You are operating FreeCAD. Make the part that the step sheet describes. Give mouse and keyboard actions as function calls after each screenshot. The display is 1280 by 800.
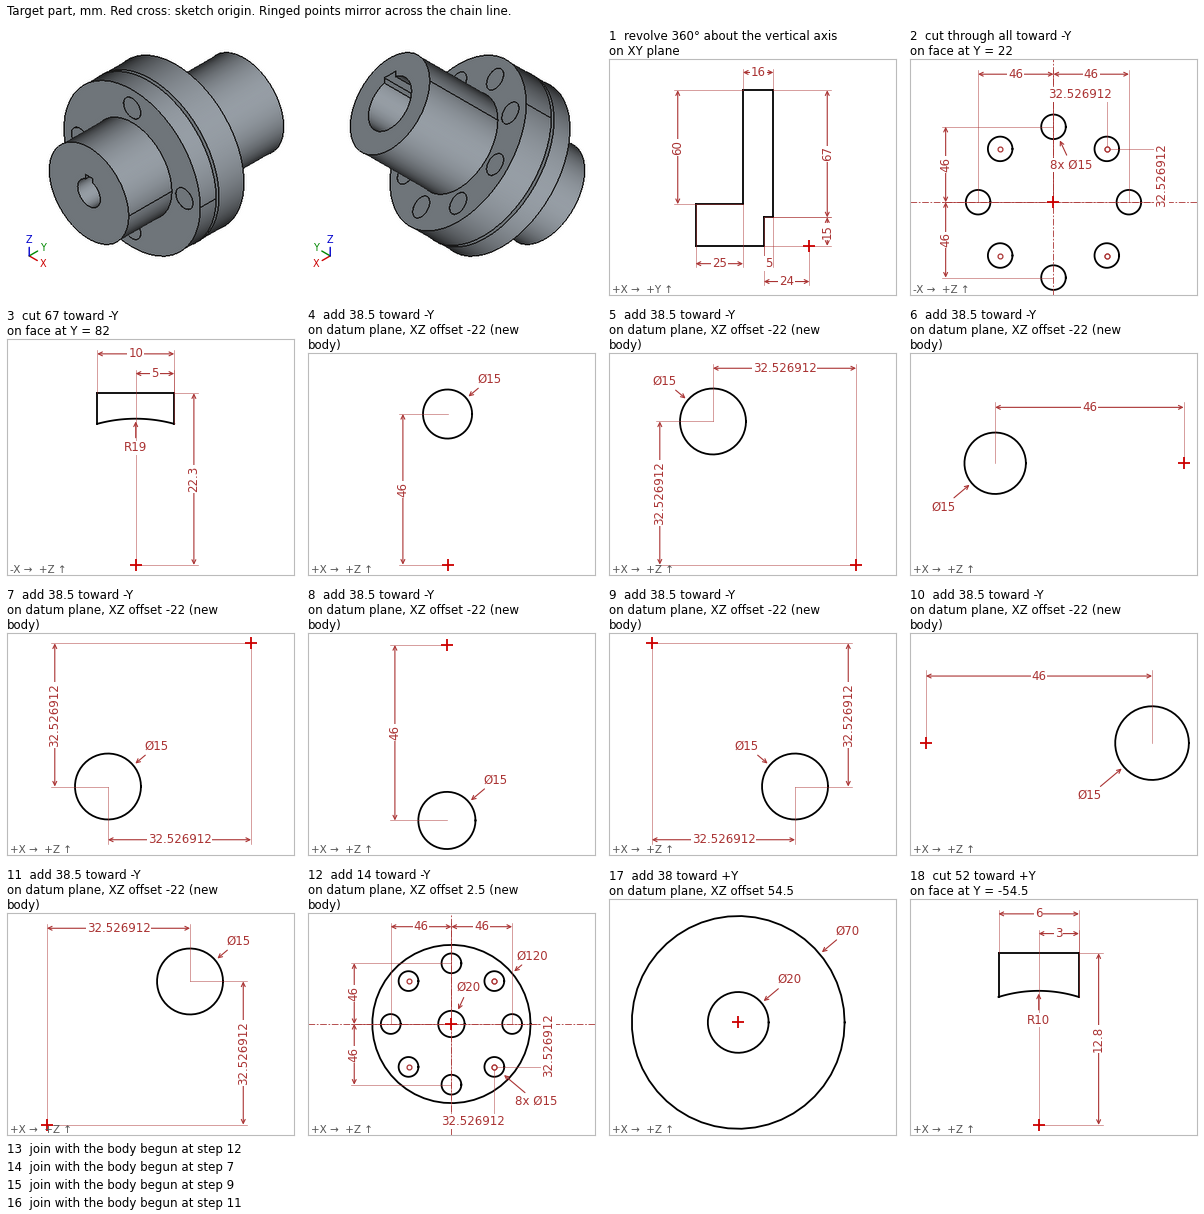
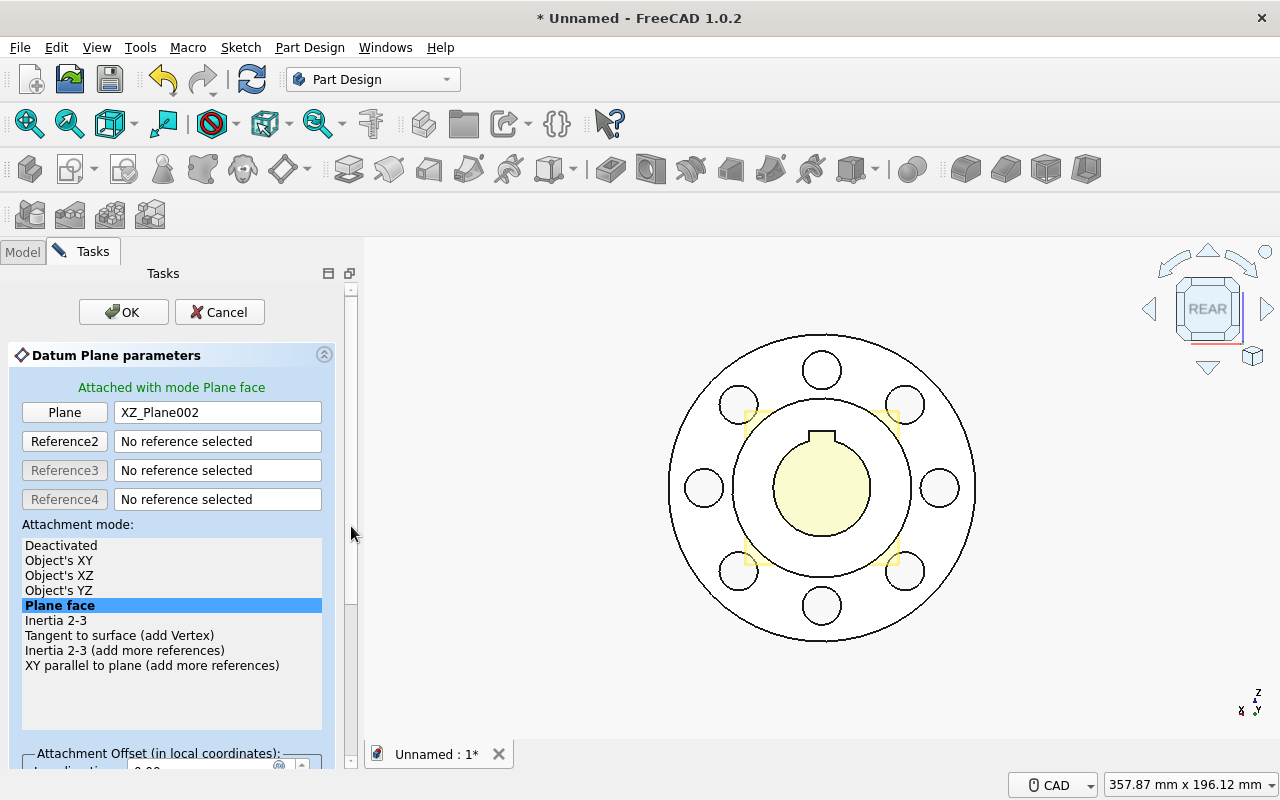
click(124, 312)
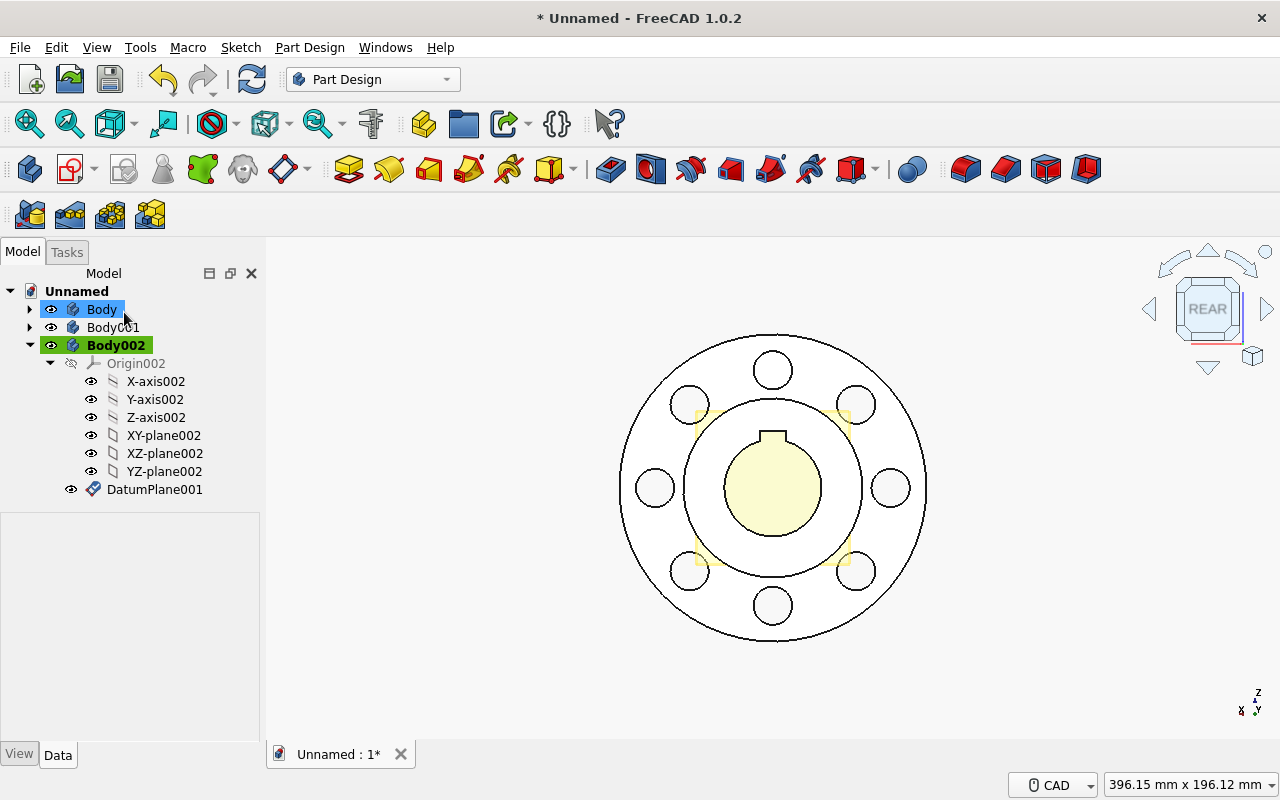
click(116, 489)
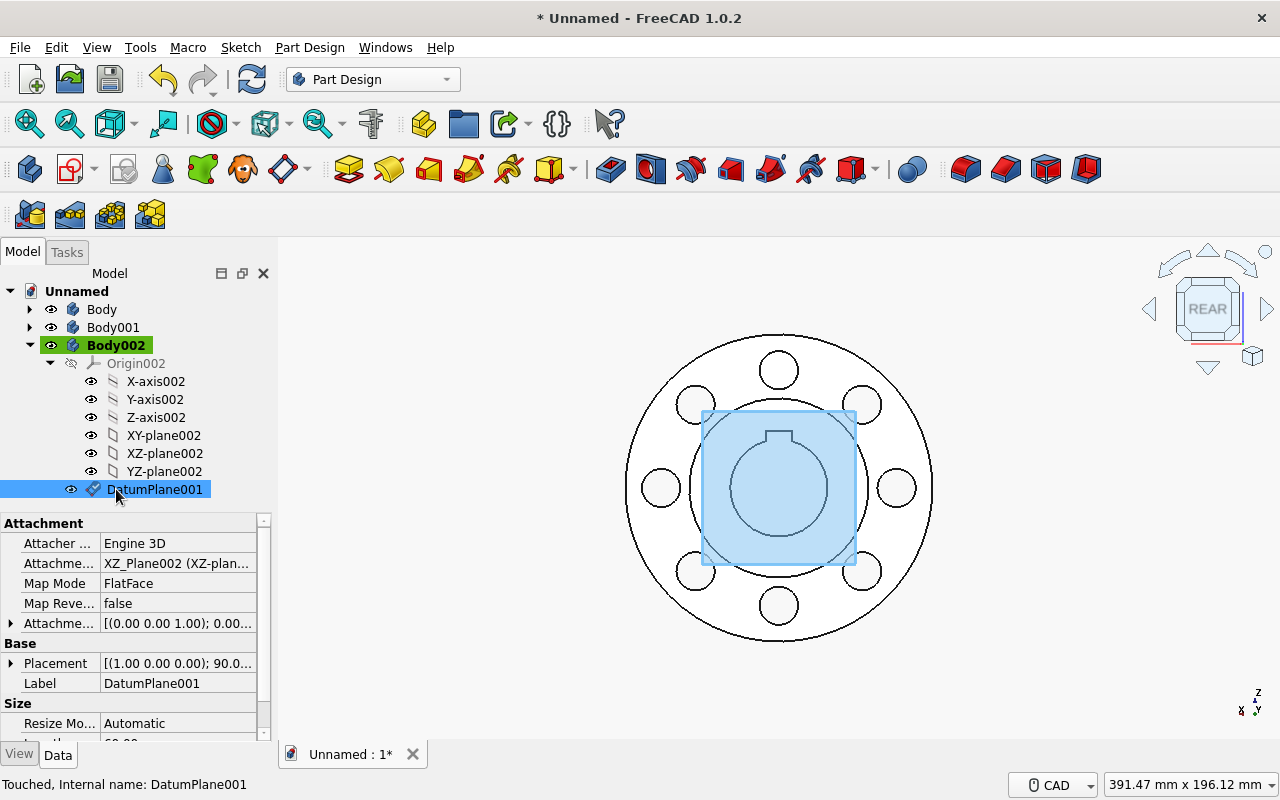
click(70, 170)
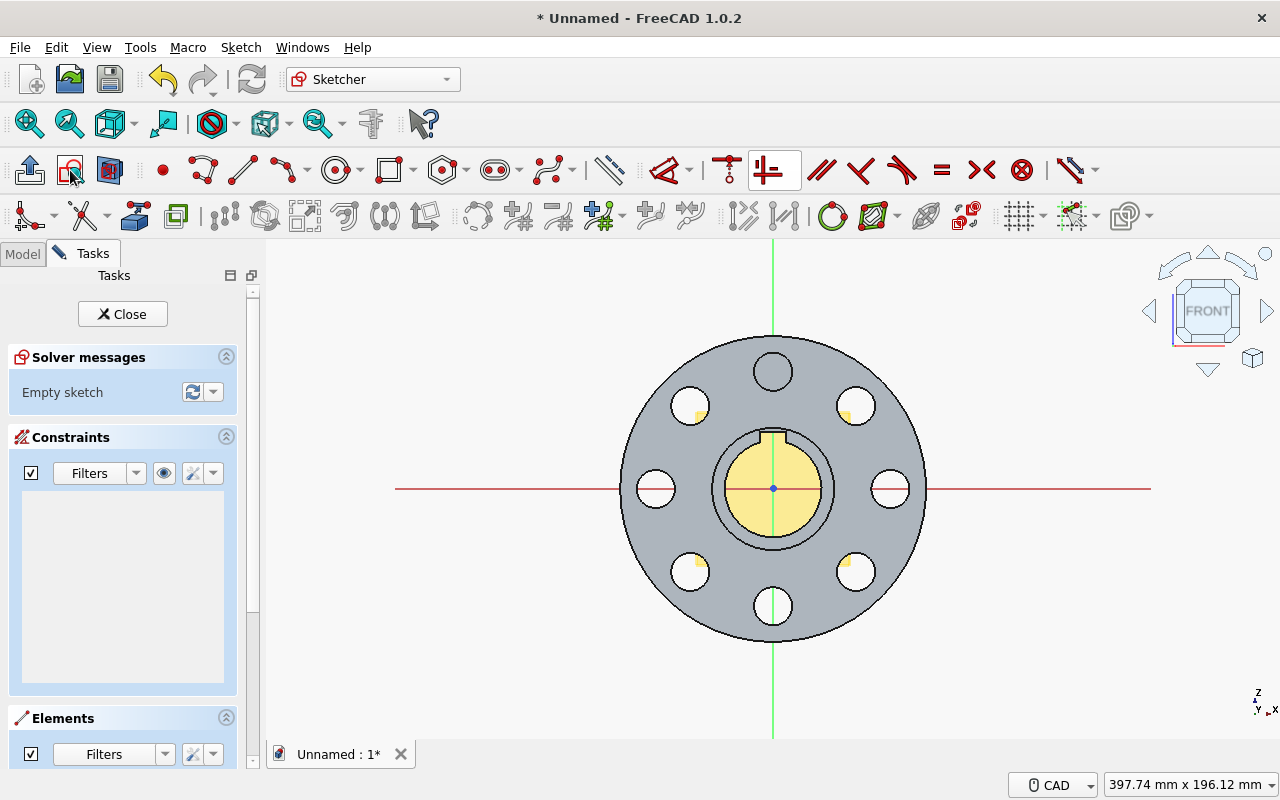
scroll(688, 396, up, 11)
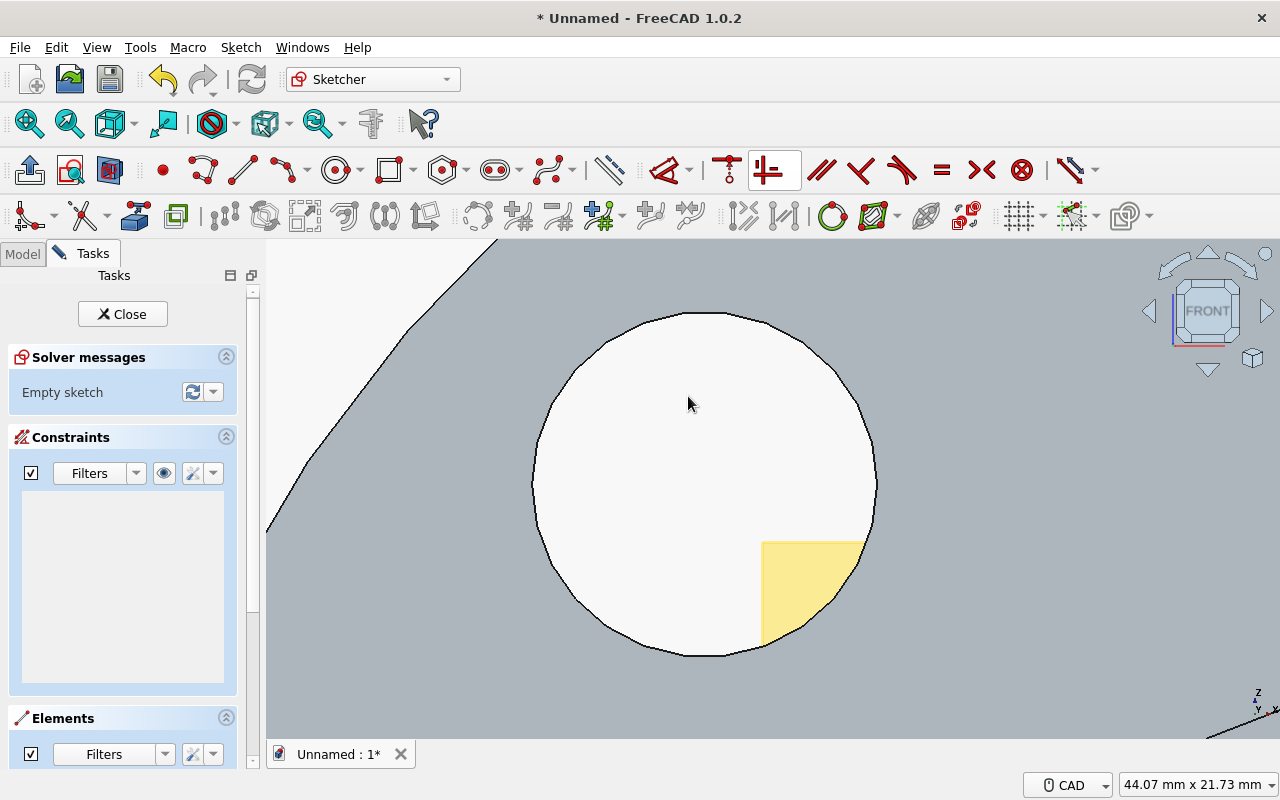
click(336, 170)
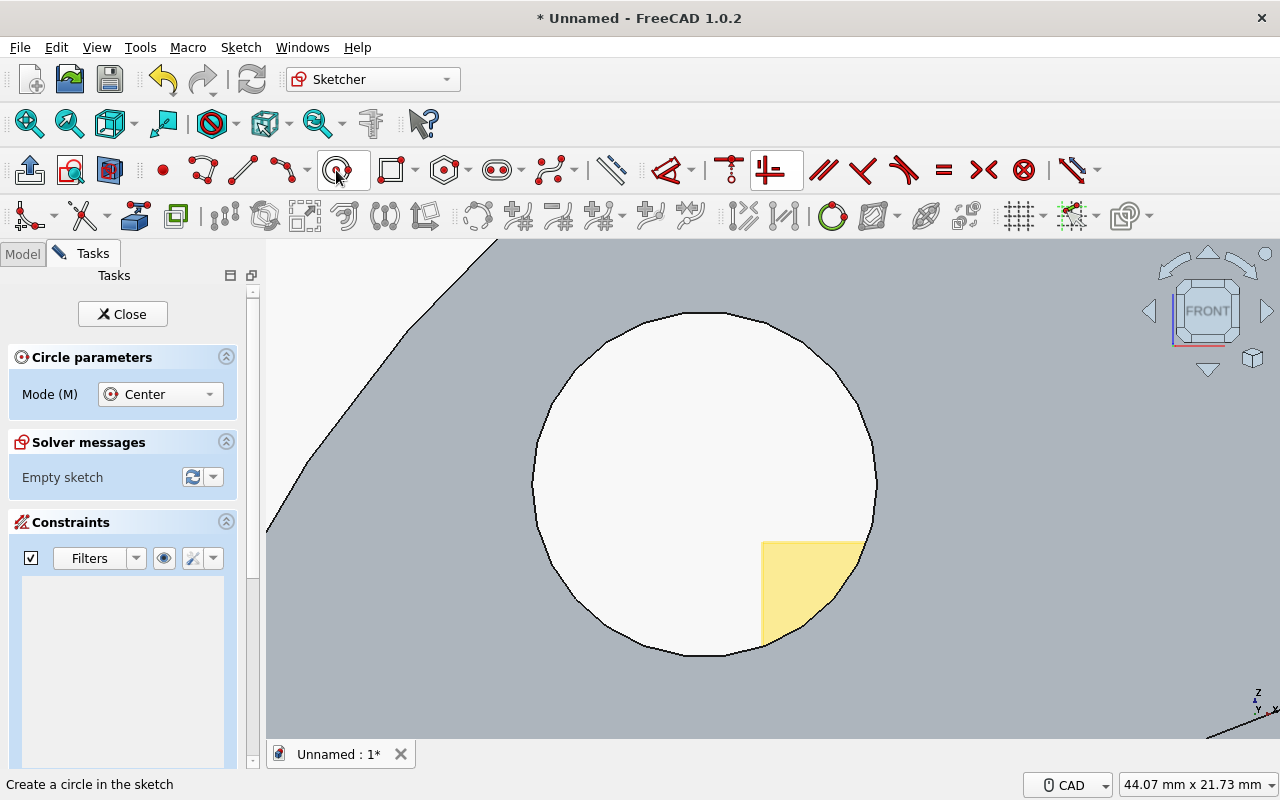
click(705, 484)
click(827, 362)
key(Escape)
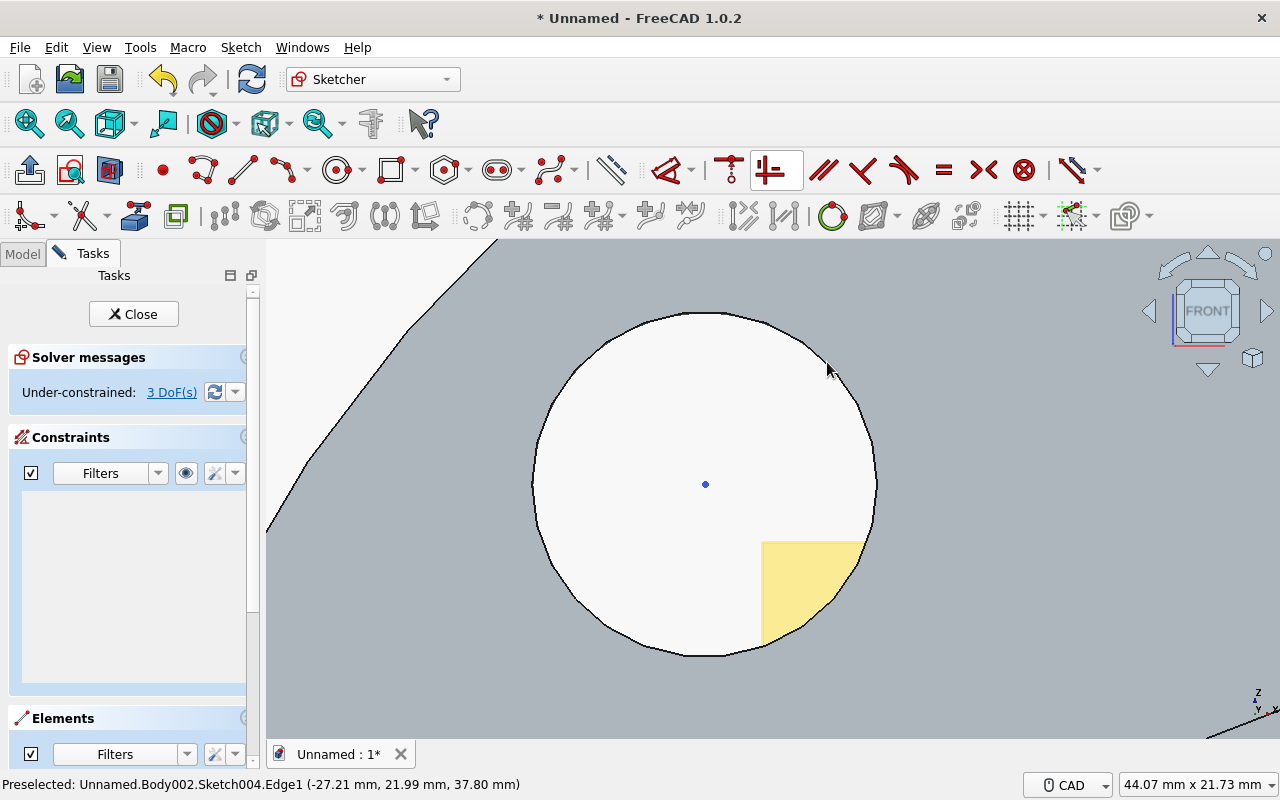
click(666, 170)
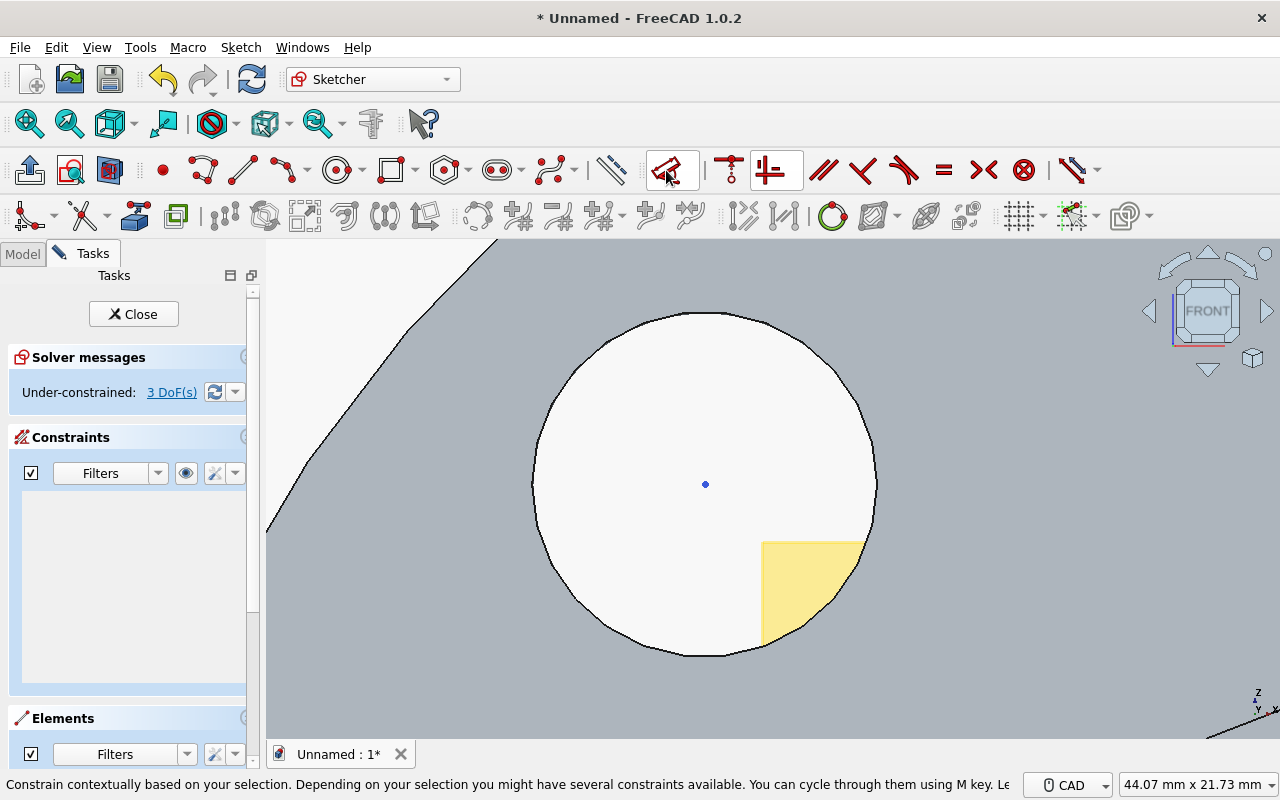
click(827, 363)
click(850, 340)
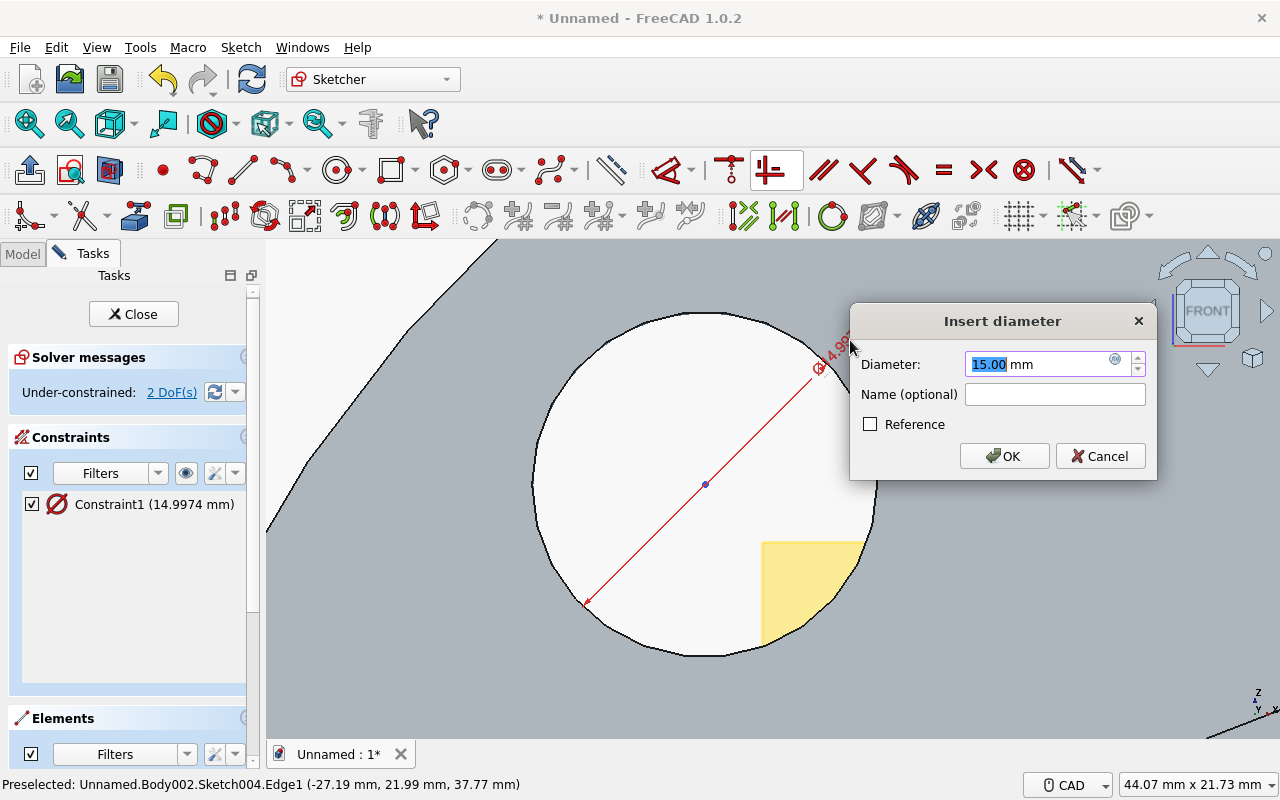
text(15)
key(Return)